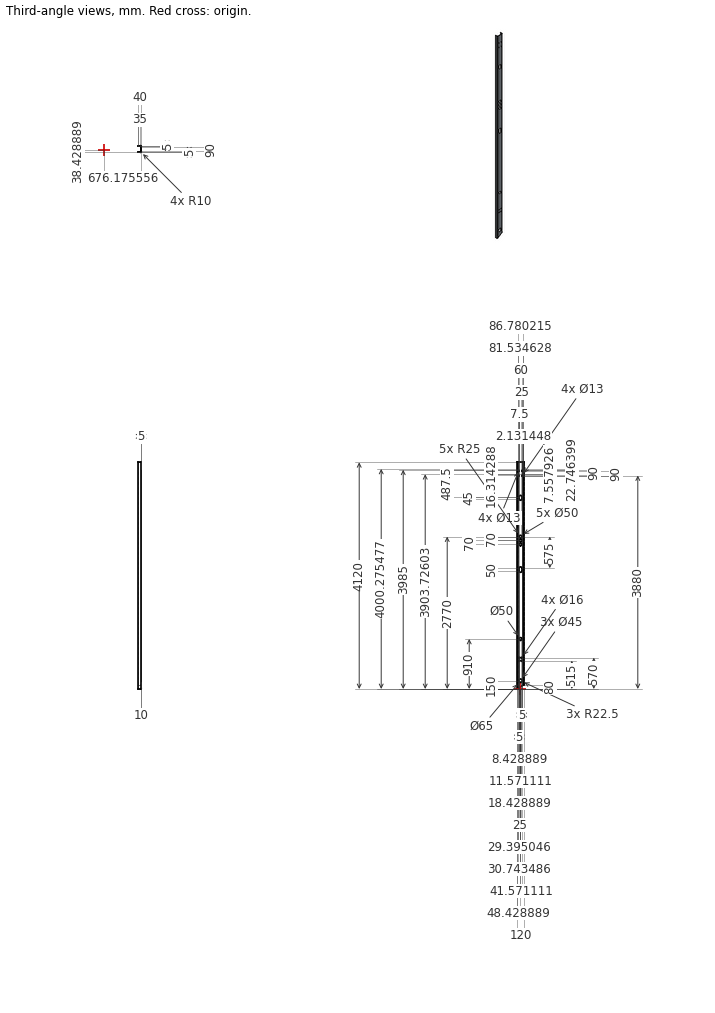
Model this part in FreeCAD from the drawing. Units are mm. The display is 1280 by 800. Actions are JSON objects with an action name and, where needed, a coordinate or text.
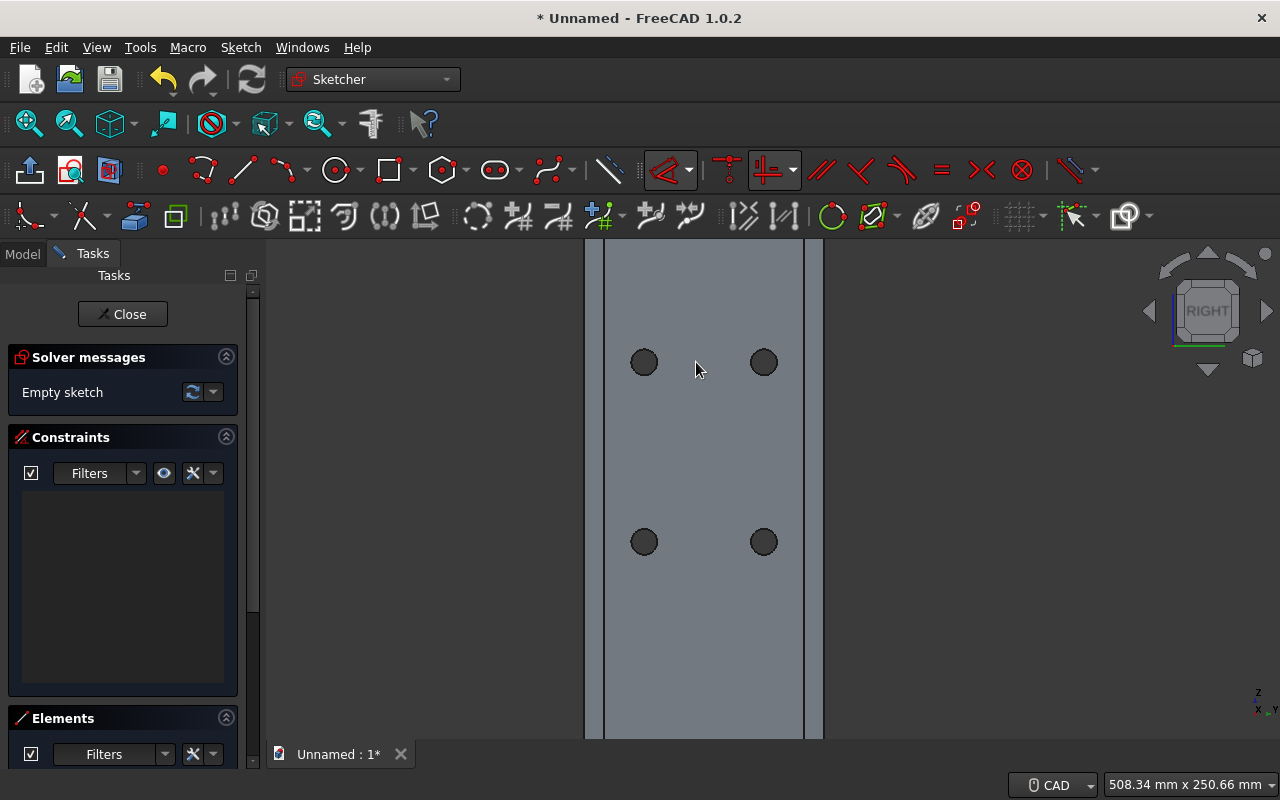
{"action": "scroll", "coordinate": [703, 468], "scroll_direction": "up", "scroll_amount": 2}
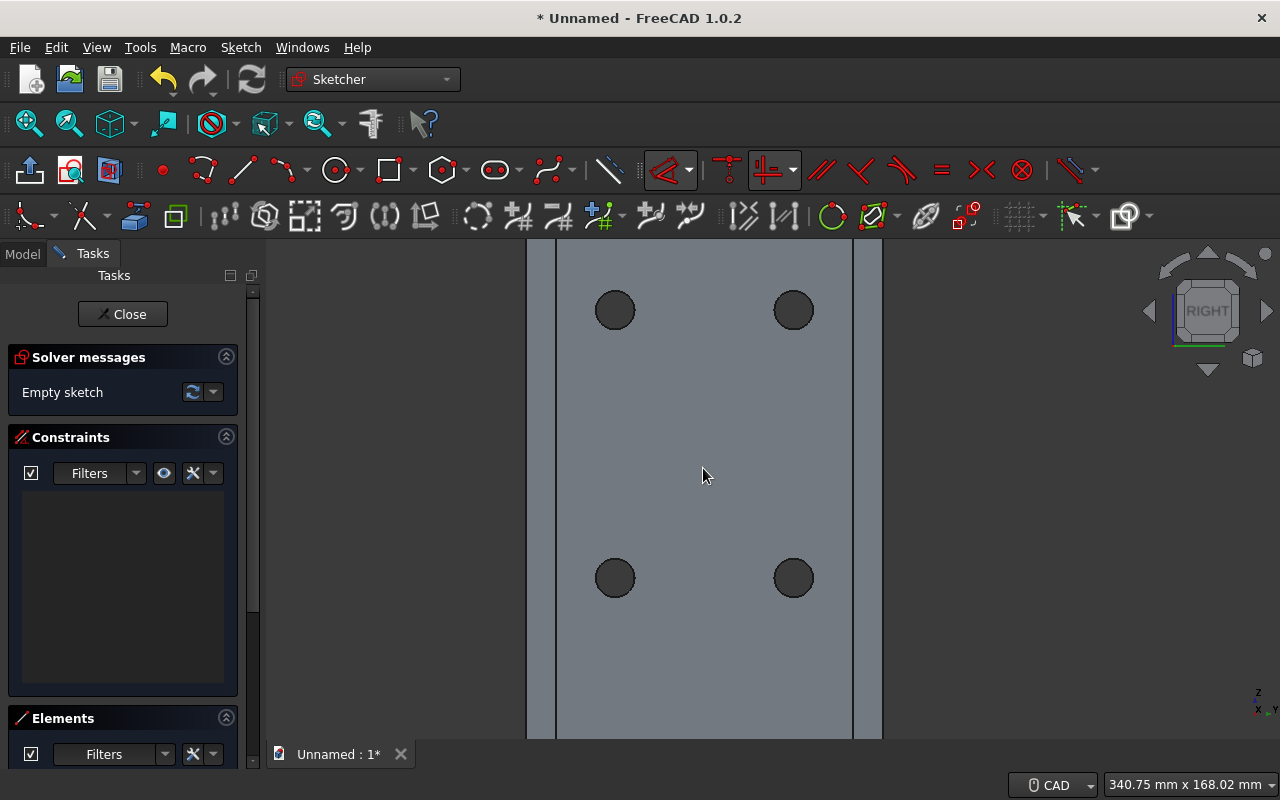
{"action": "left_click", "coordinate": [336, 170]}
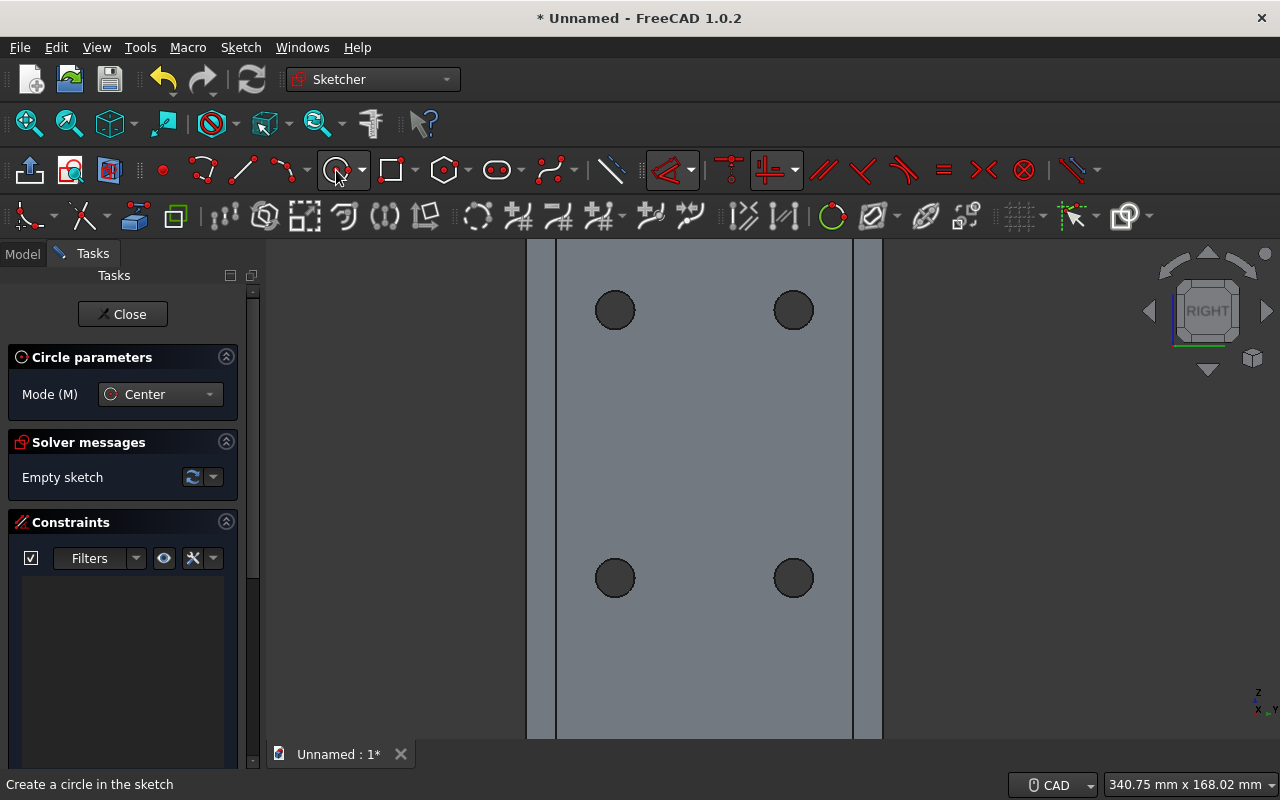
{"action": "left_click", "coordinate": [794, 623]}
{"action": "mouse_move", "coordinate": [807, 609]}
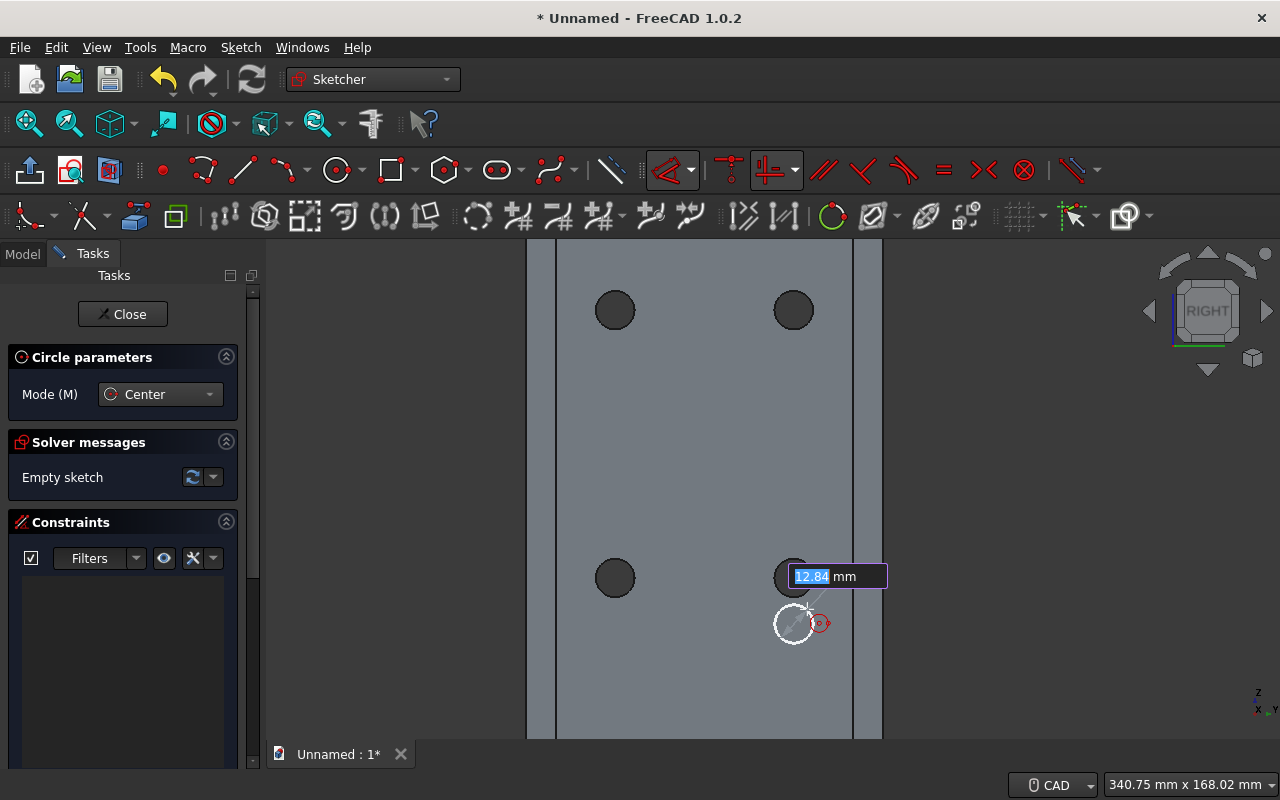
{"action": "type", "text": "13"}
{"action": "key", "text": "Return"}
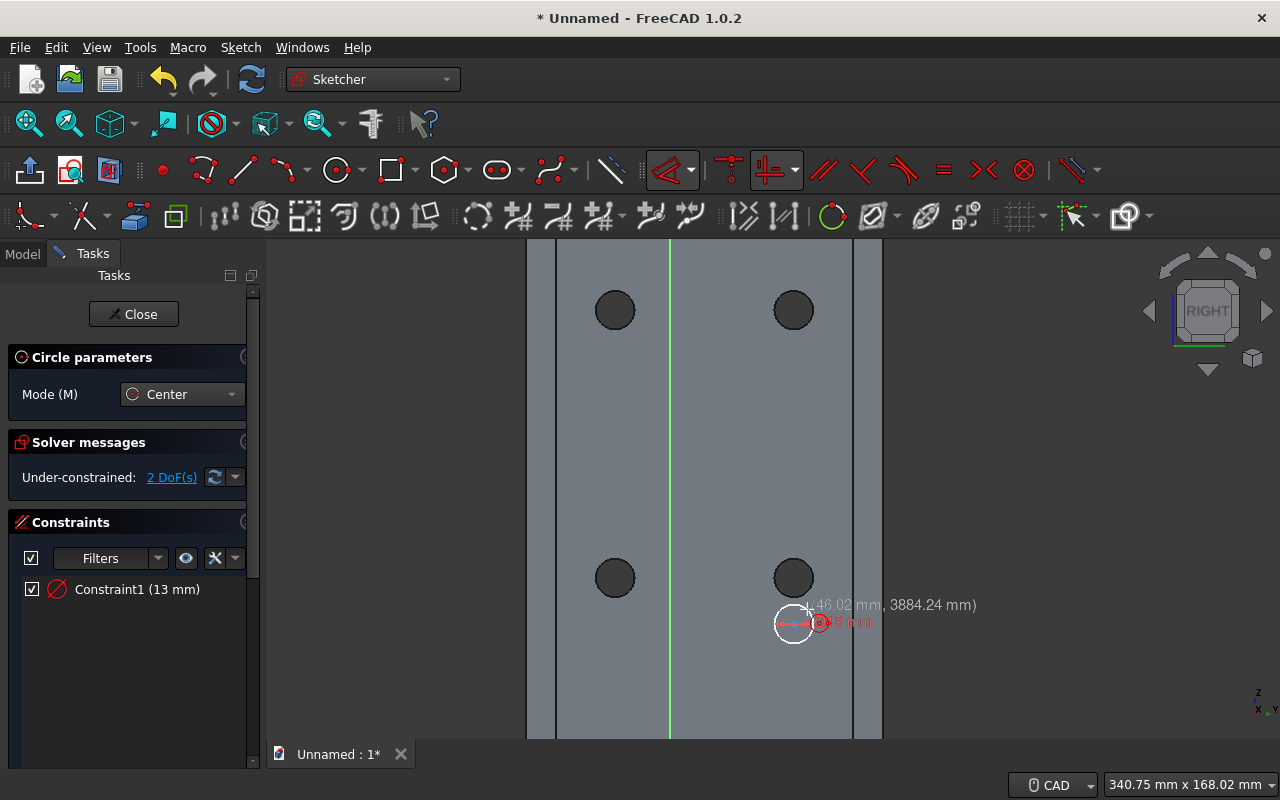
{"action": "left_click", "coordinate": [794, 355]}
{"action": "mouse_move", "coordinate": [807, 341]}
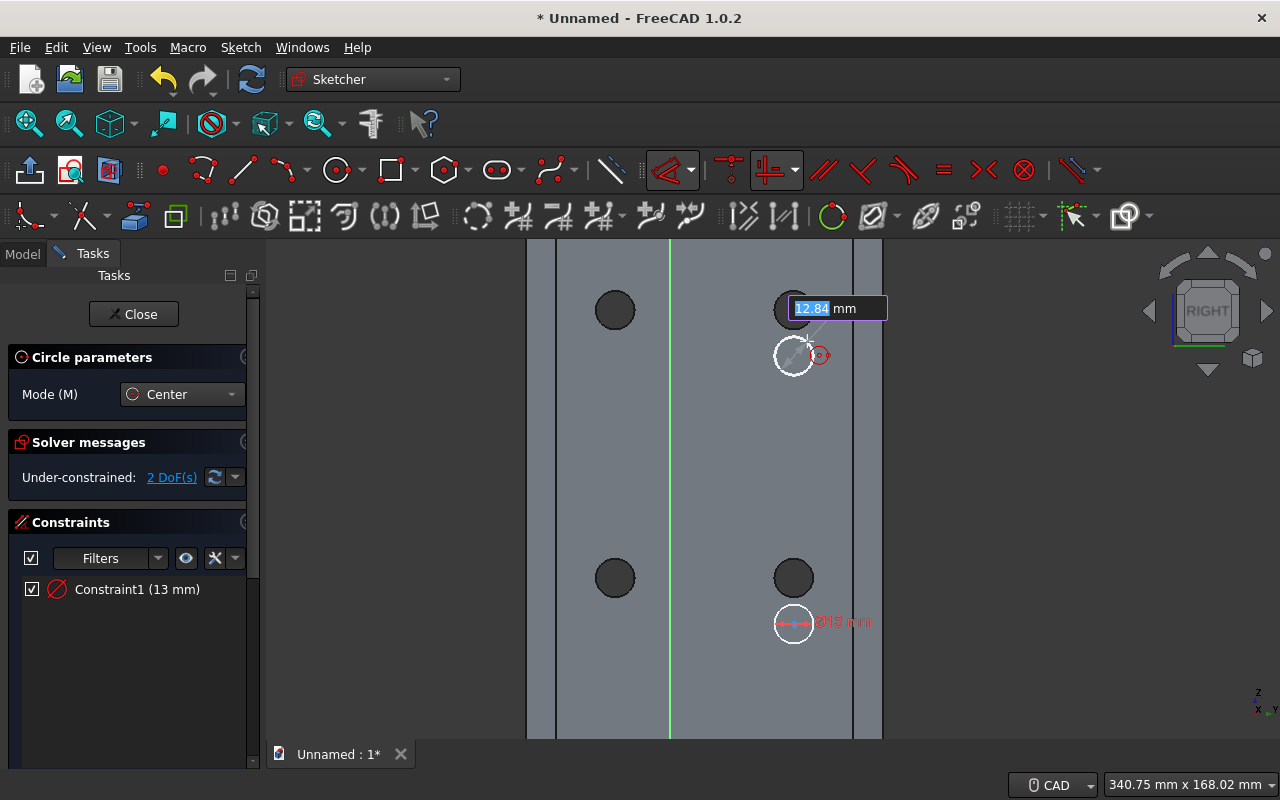
{"action": "type", "text": "13"}
{"action": "key", "text": "Return"}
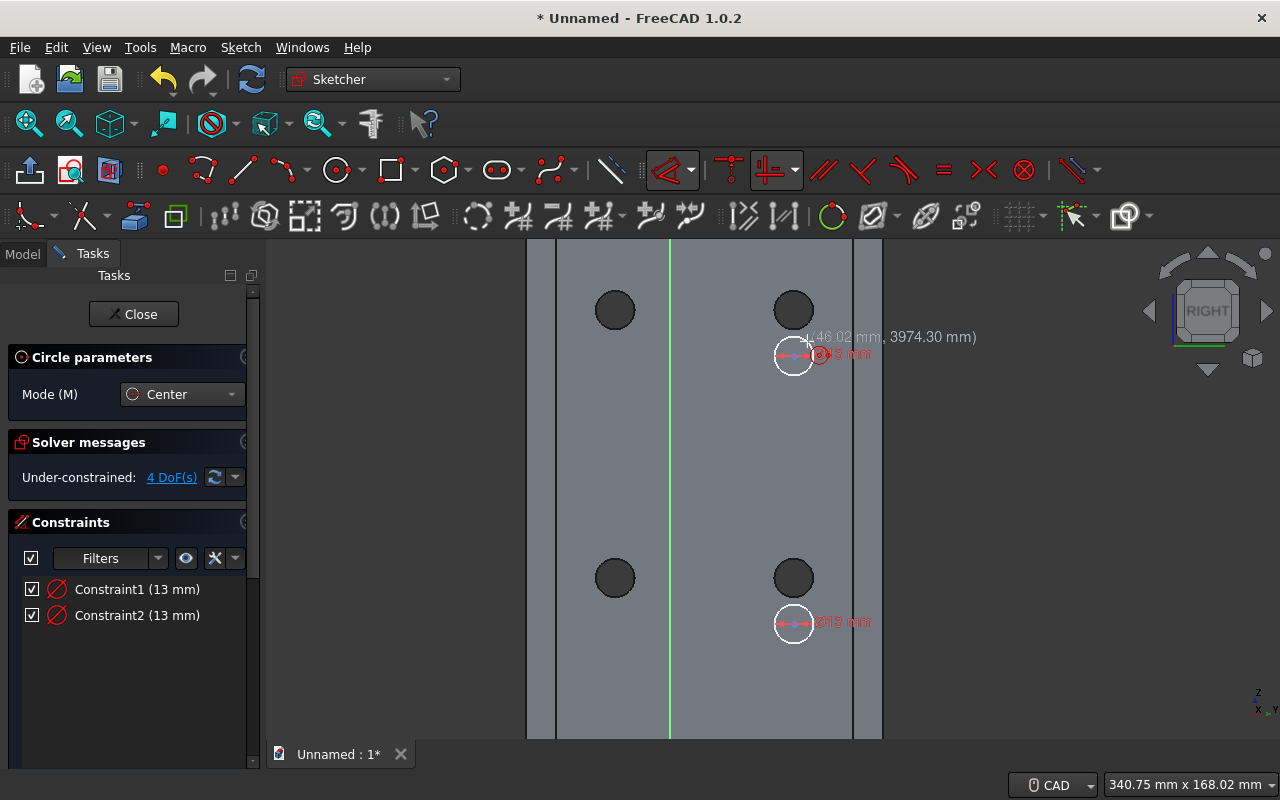
{"action": "left_click", "coordinate": [615, 355]}
{"action": "mouse_move", "coordinate": [629, 341]}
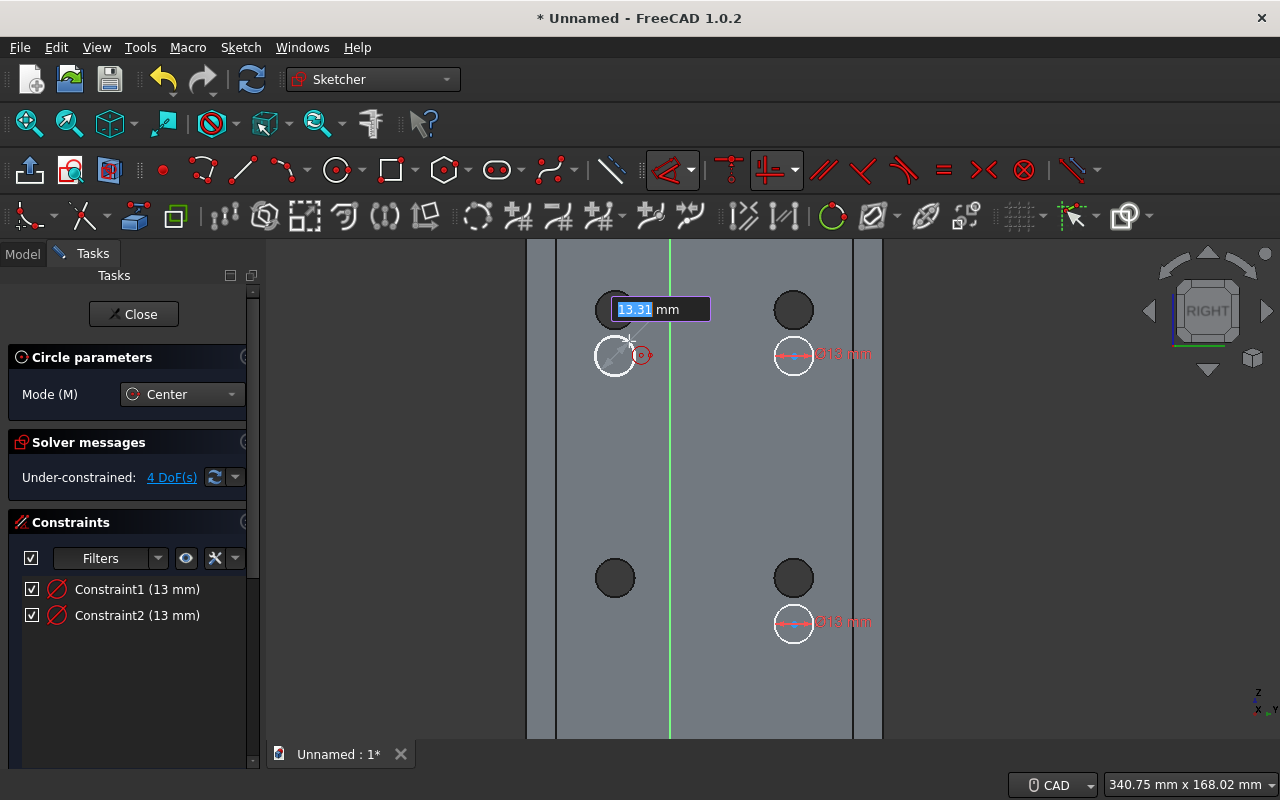
{"action": "type", "text": "13"}
{"action": "key", "text": "Return"}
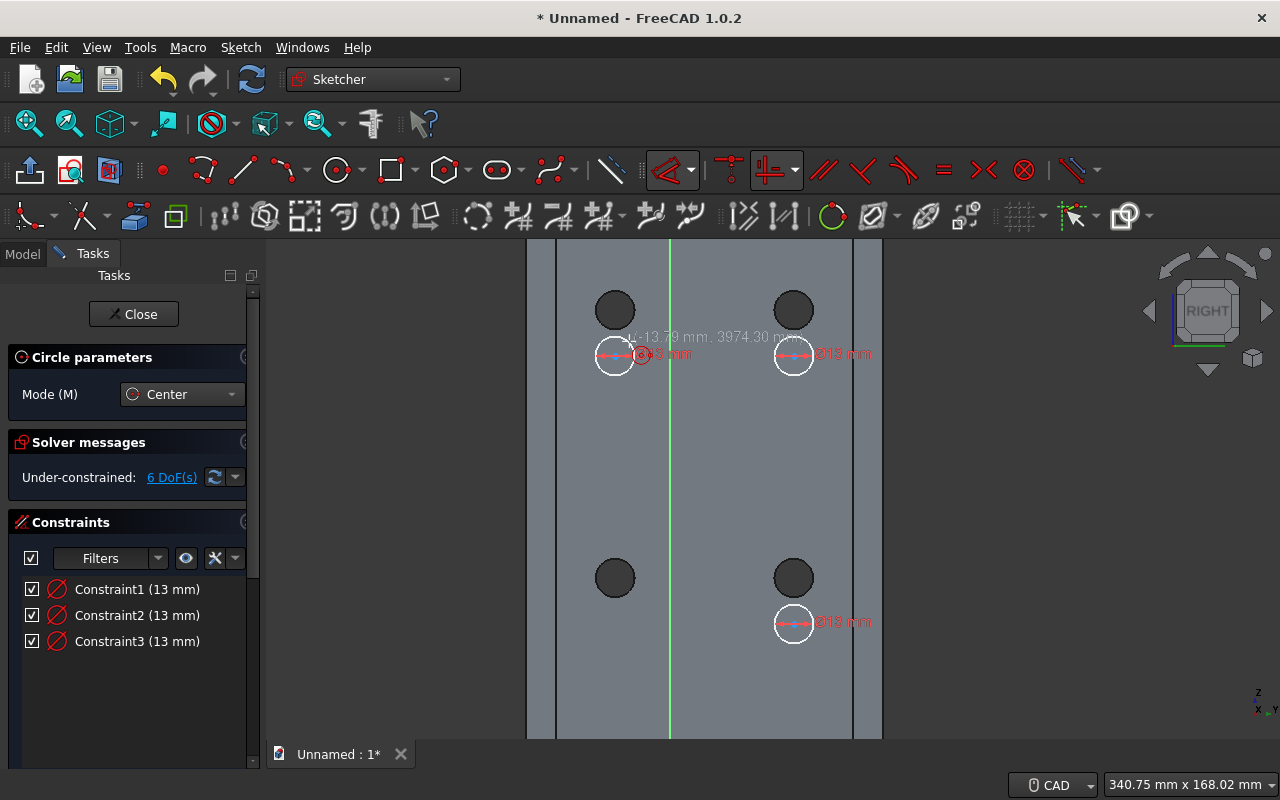
{"action": "left_click", "coordinate": [615, 623]}
{"action": "mouse_move", "coordinate": [629, 609]}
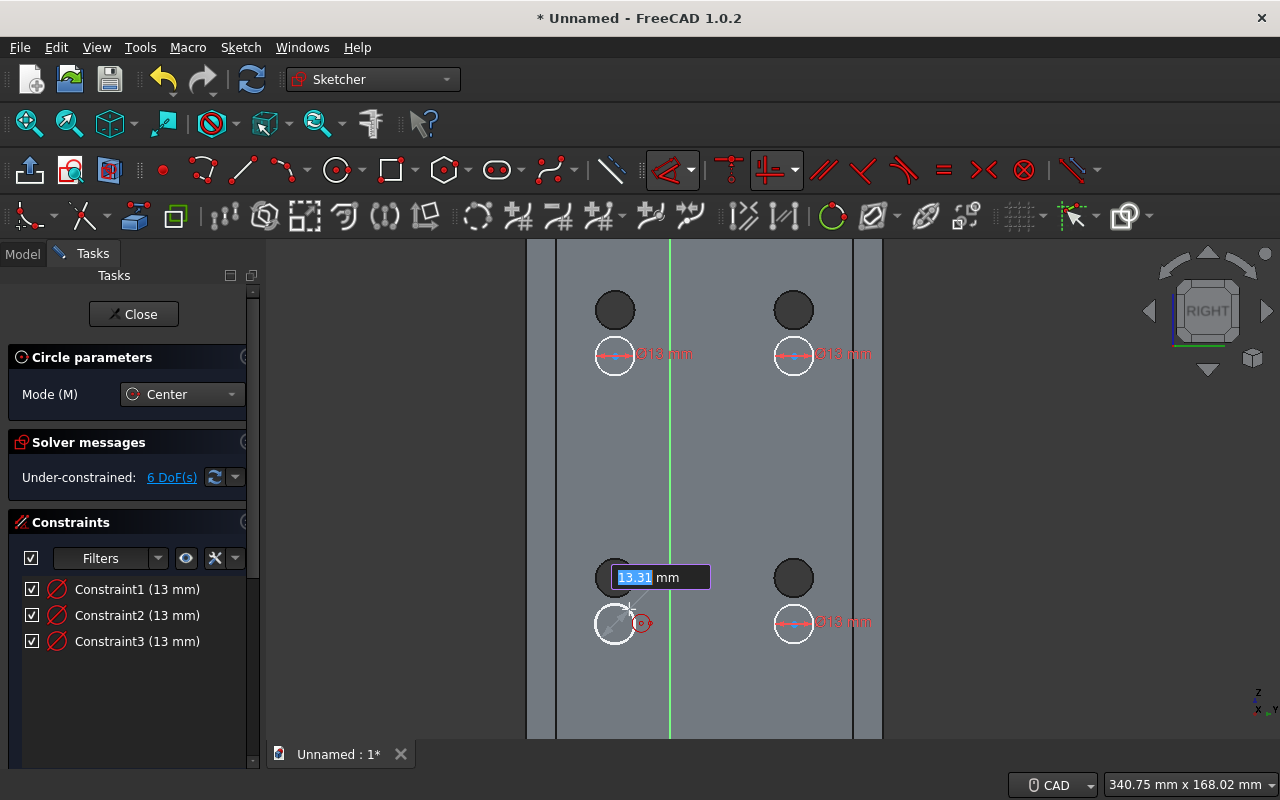
{"action": "type", "text": "13"}
{"action": "key", "text": "Return"}
{"action": "key", "text": "Escape"}